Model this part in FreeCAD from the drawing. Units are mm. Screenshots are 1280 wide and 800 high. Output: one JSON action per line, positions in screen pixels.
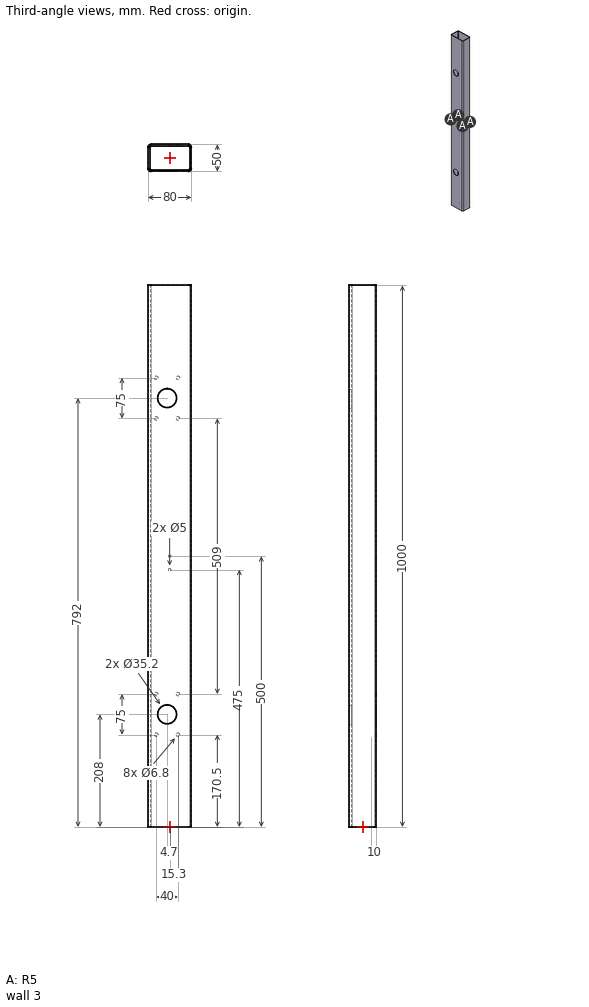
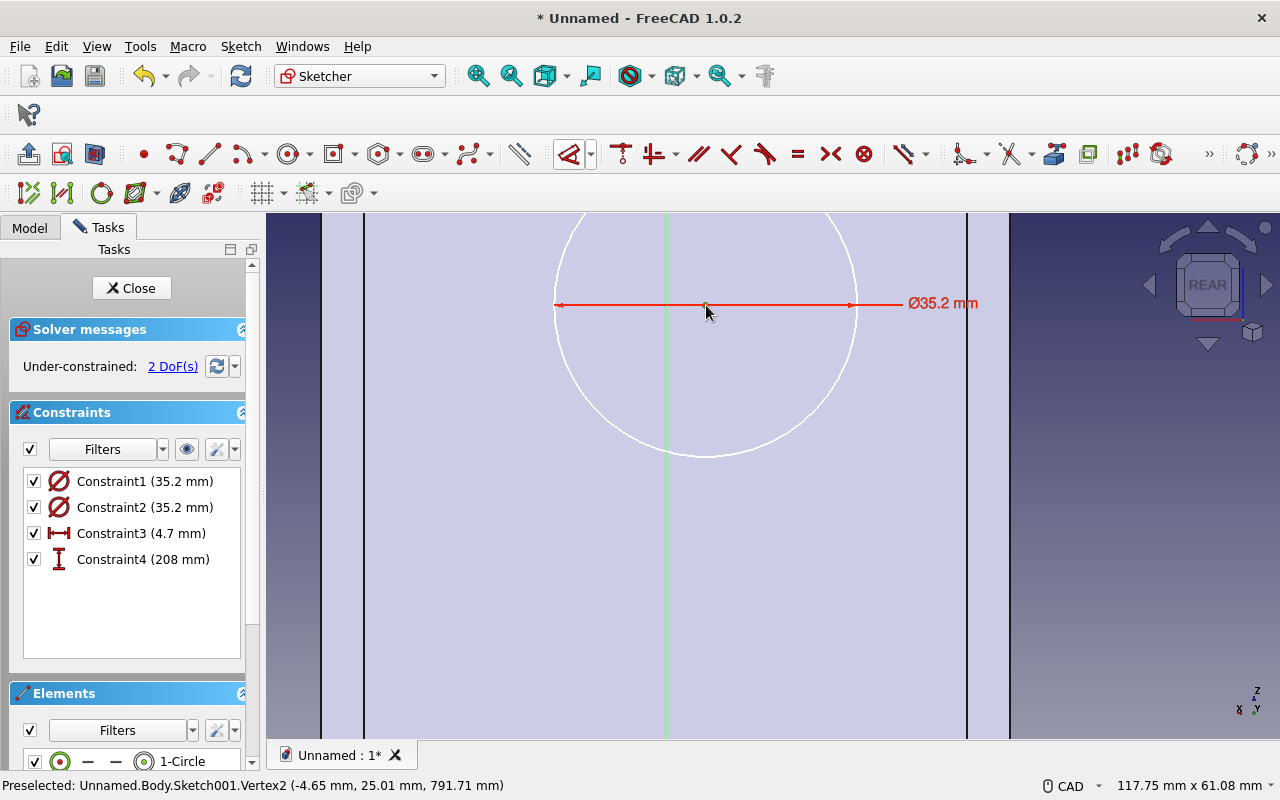
{"action": "key", "text": "l"}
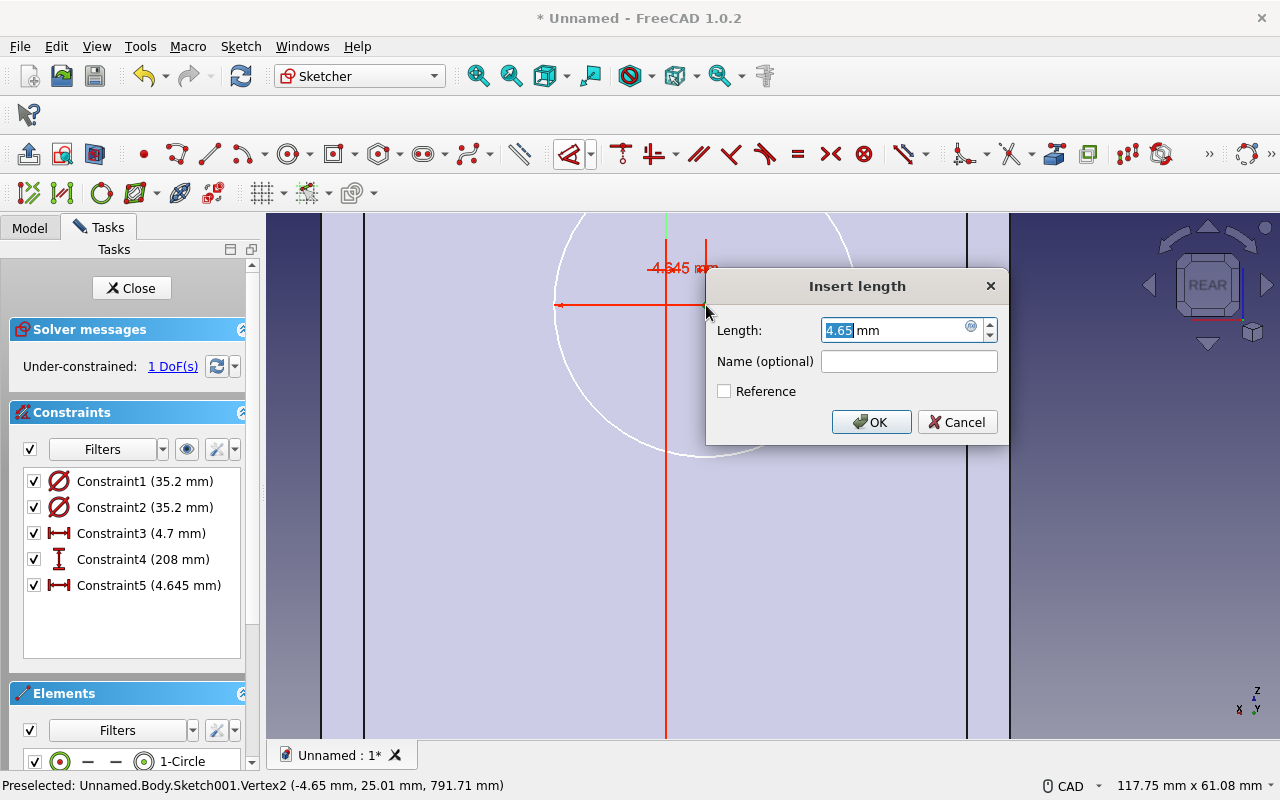
{"action": "type", "text": "4.7"}
{"action": "key", "text": "Return"}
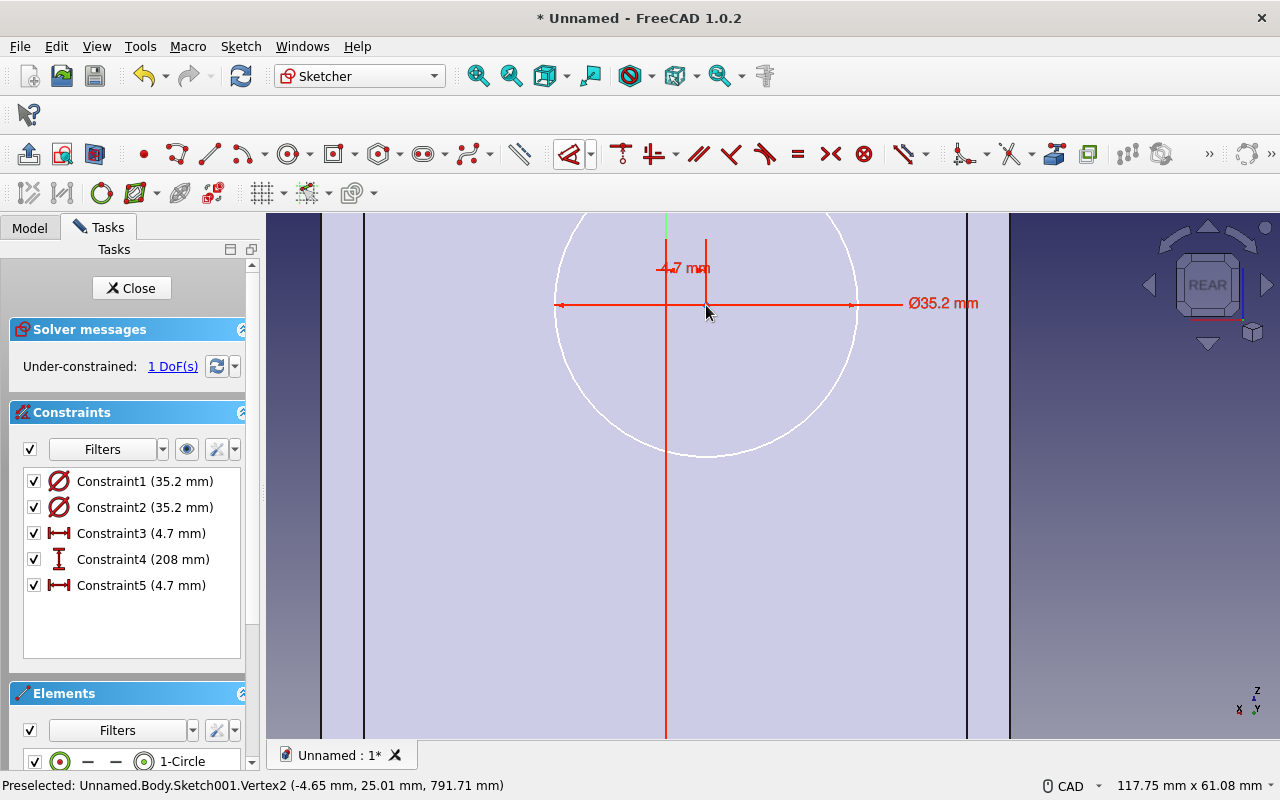
{"action": "scroll", "coordinate": [704, 310], "scroll_direction": "down", "scroll_amount": 15}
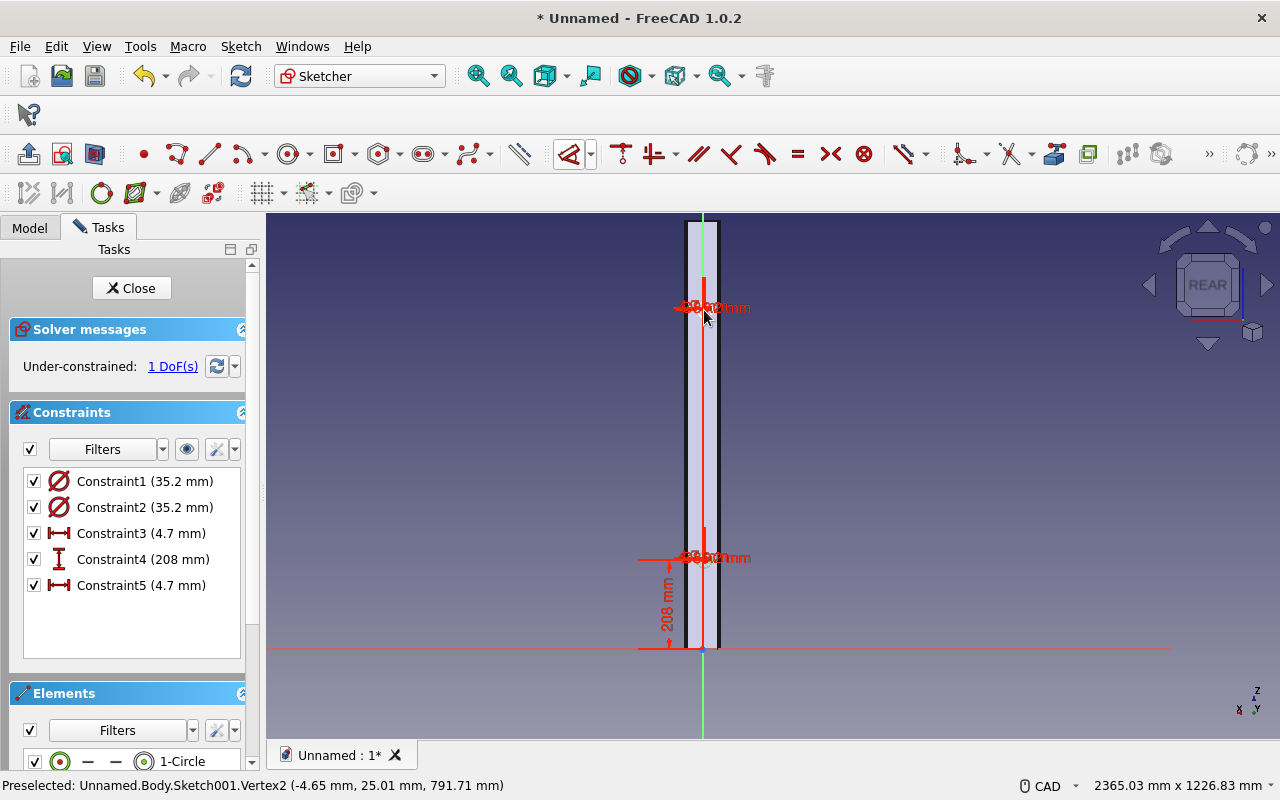
{"action": "left_click", "coordinate": [705, 310]}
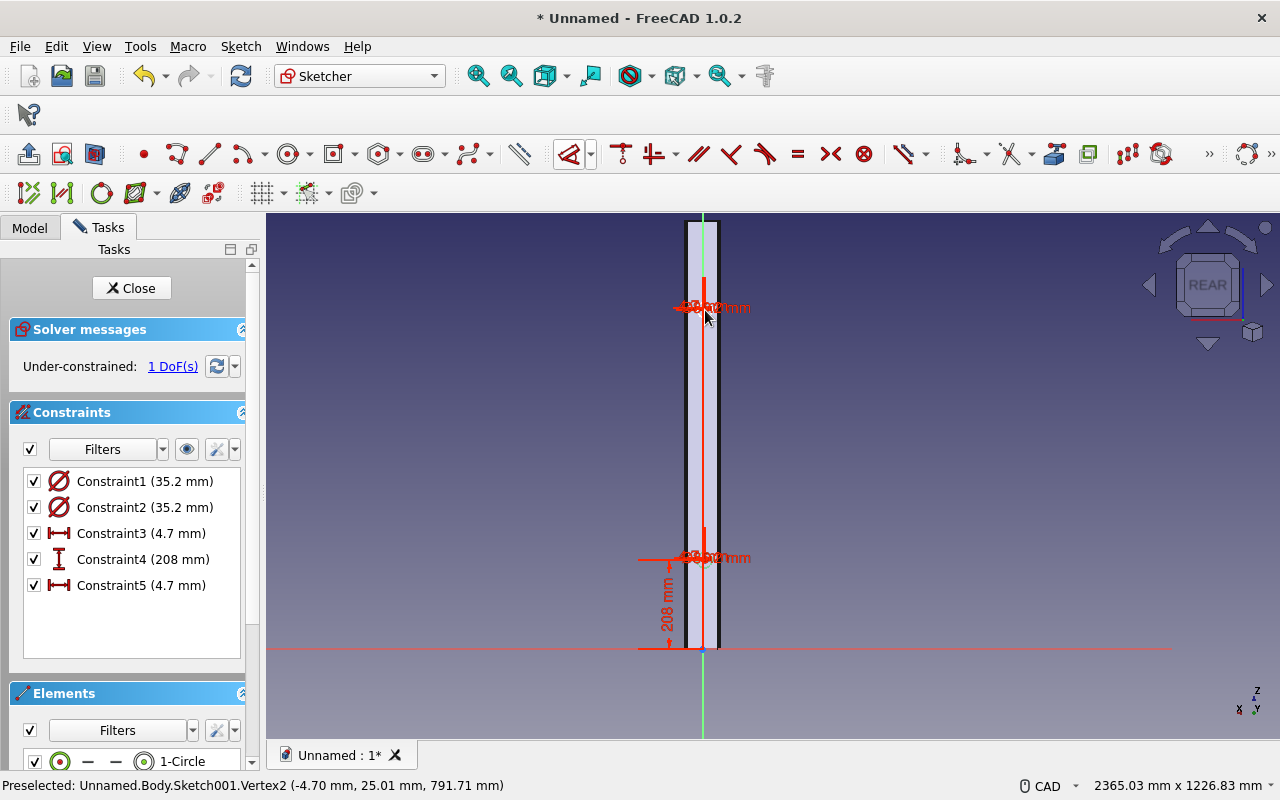
{"action": "left_click", "coordinate": [590, 154]}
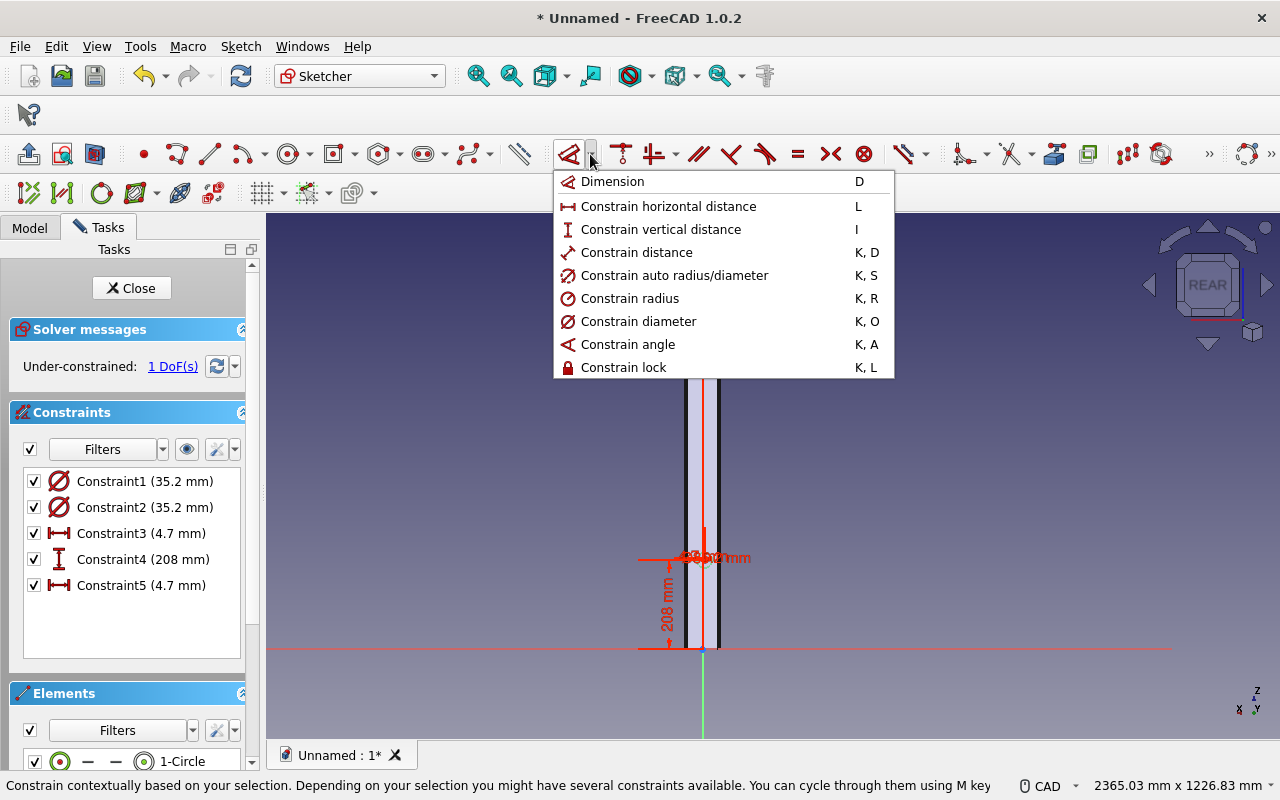
{"action": "left_click", "coordinate": [724, 230]}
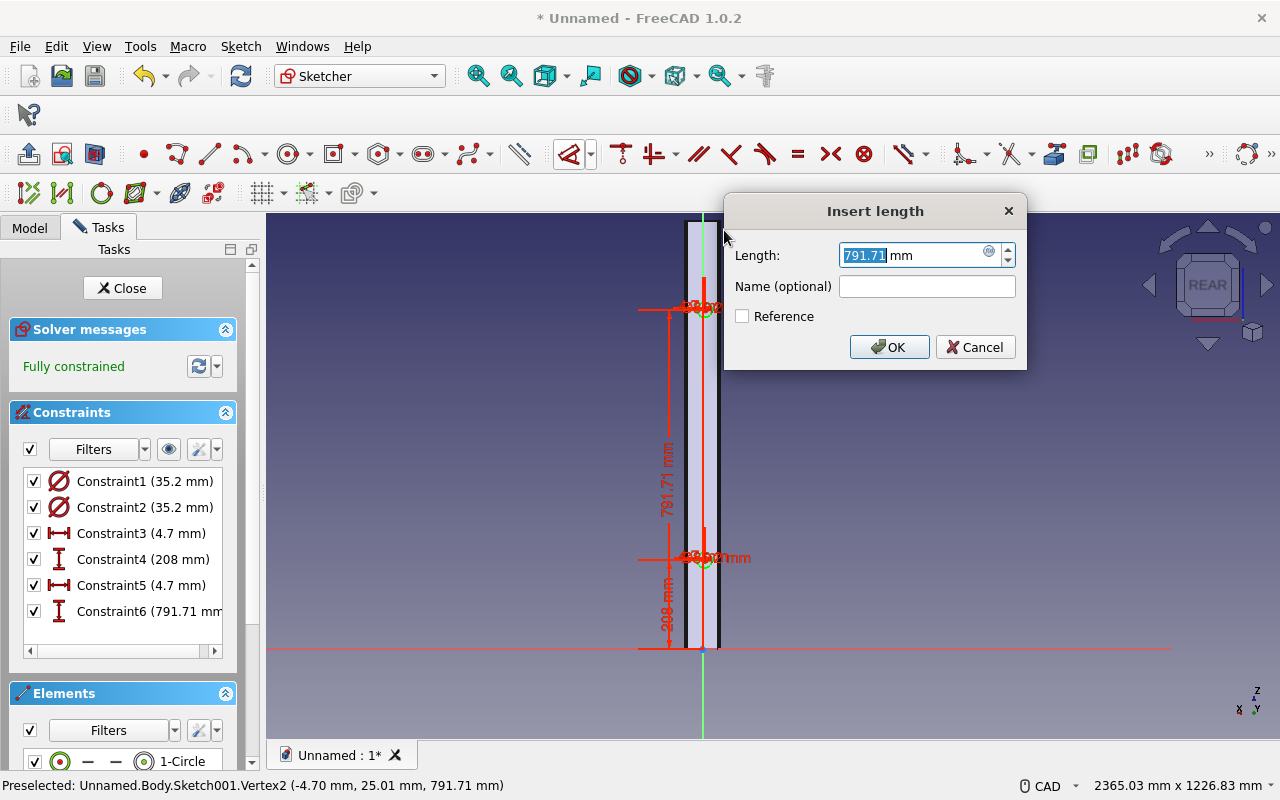
{"action": "type", "text": "792"}
{"action": "key", "text": "Return"}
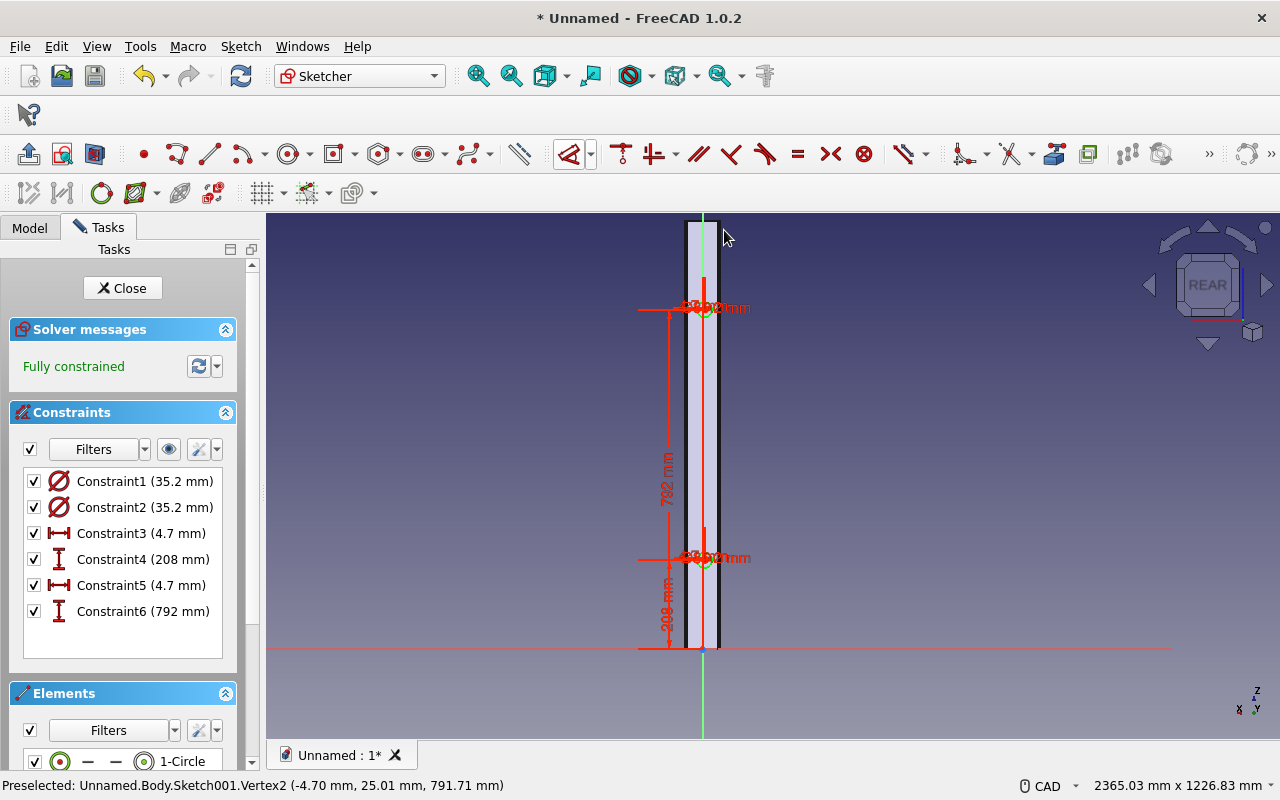
{"action": "left_click", "coordinate": [123, 288]}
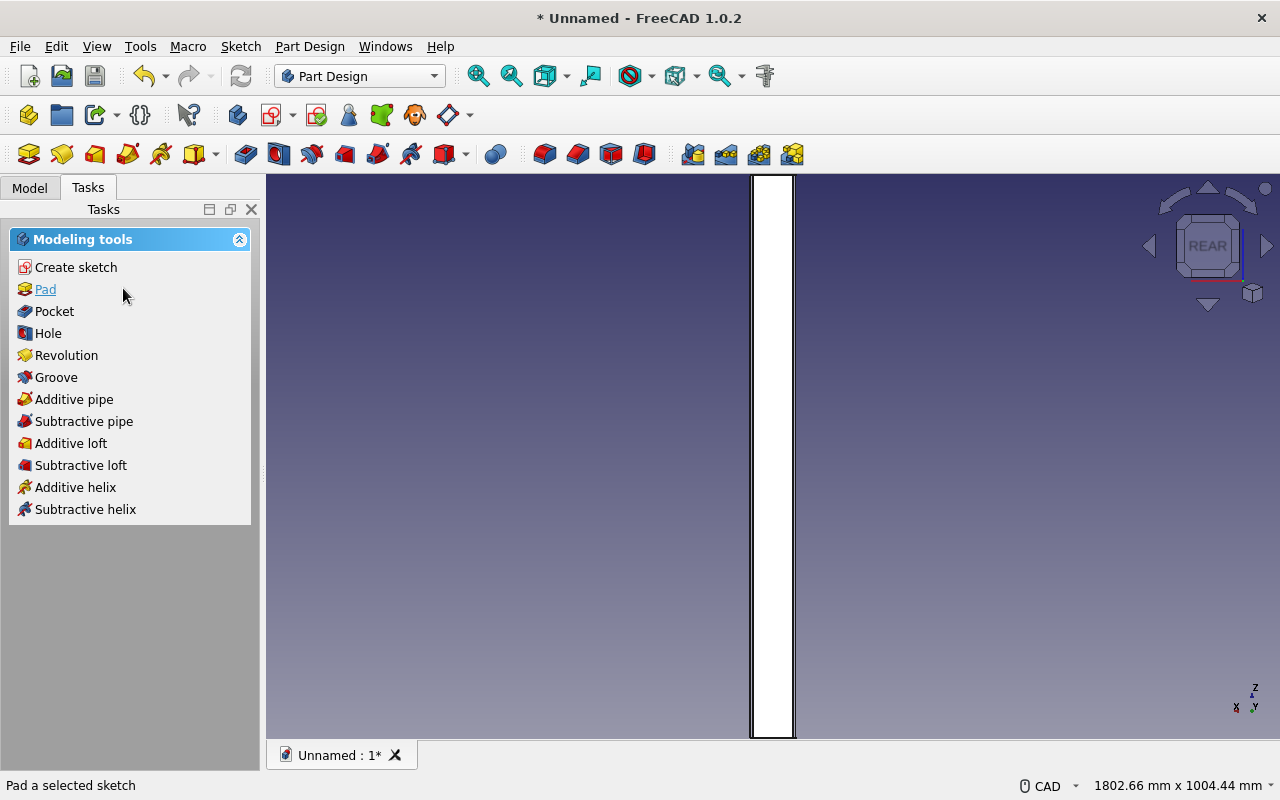
{"action": "left_click", "coordinate": [246, 154]}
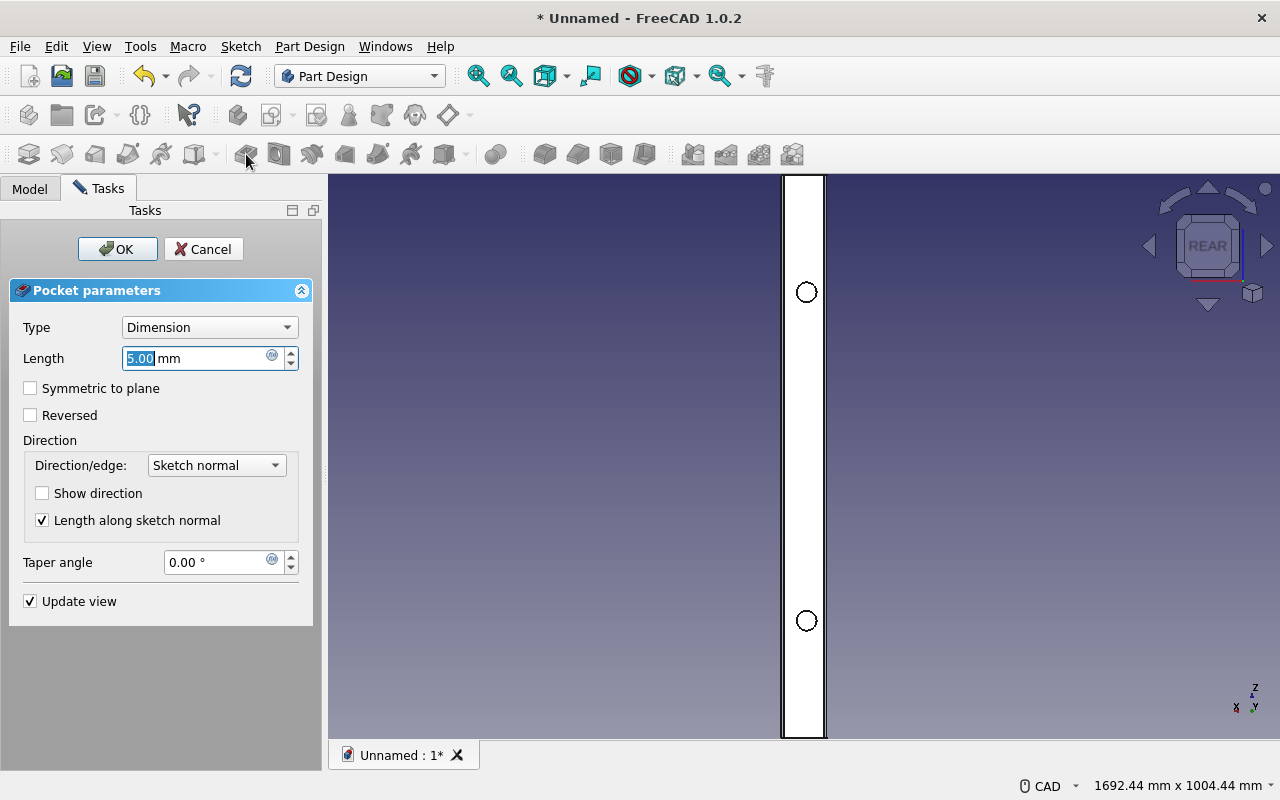
{"action": "left_click", "coordinate": [210, 328]}